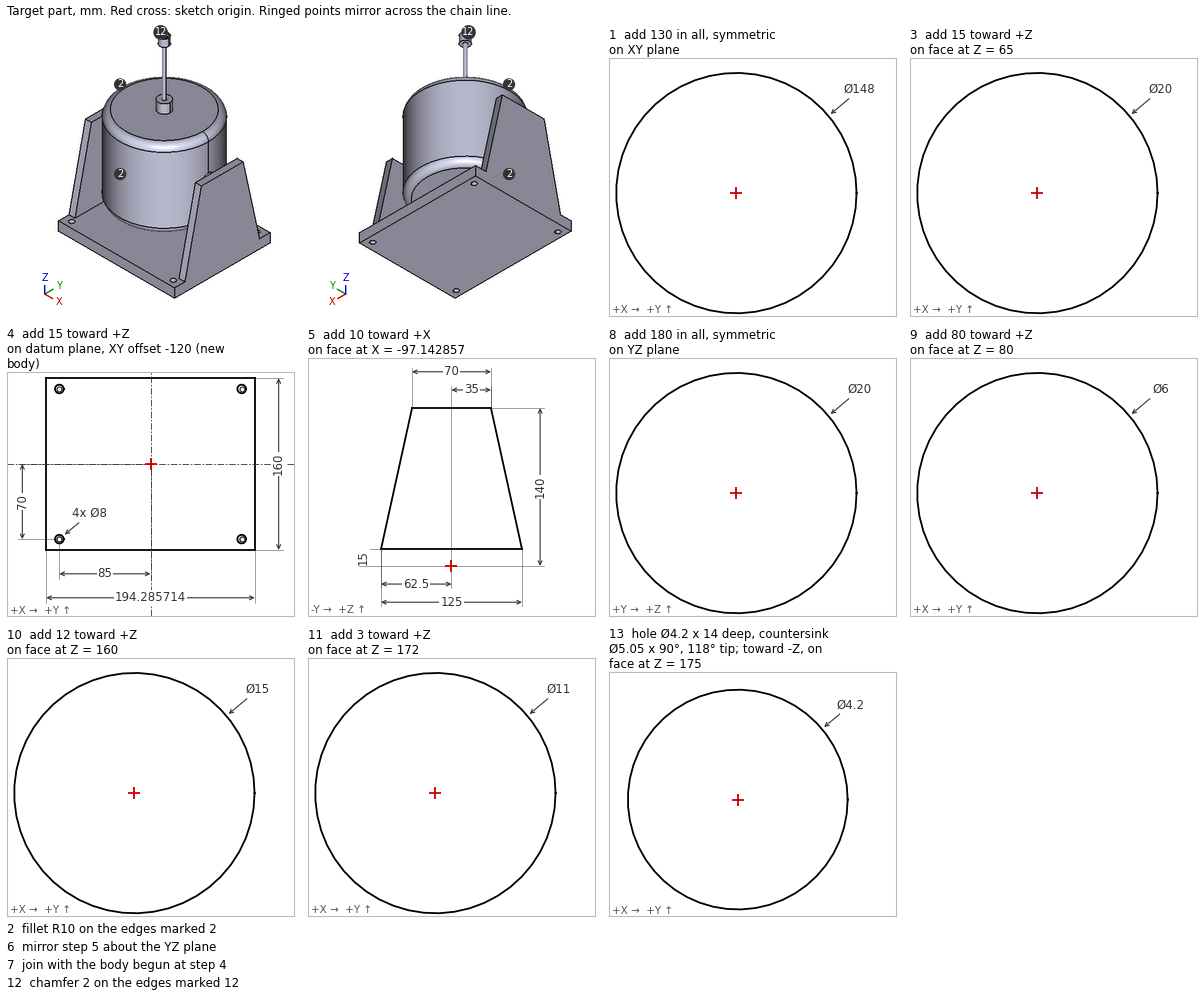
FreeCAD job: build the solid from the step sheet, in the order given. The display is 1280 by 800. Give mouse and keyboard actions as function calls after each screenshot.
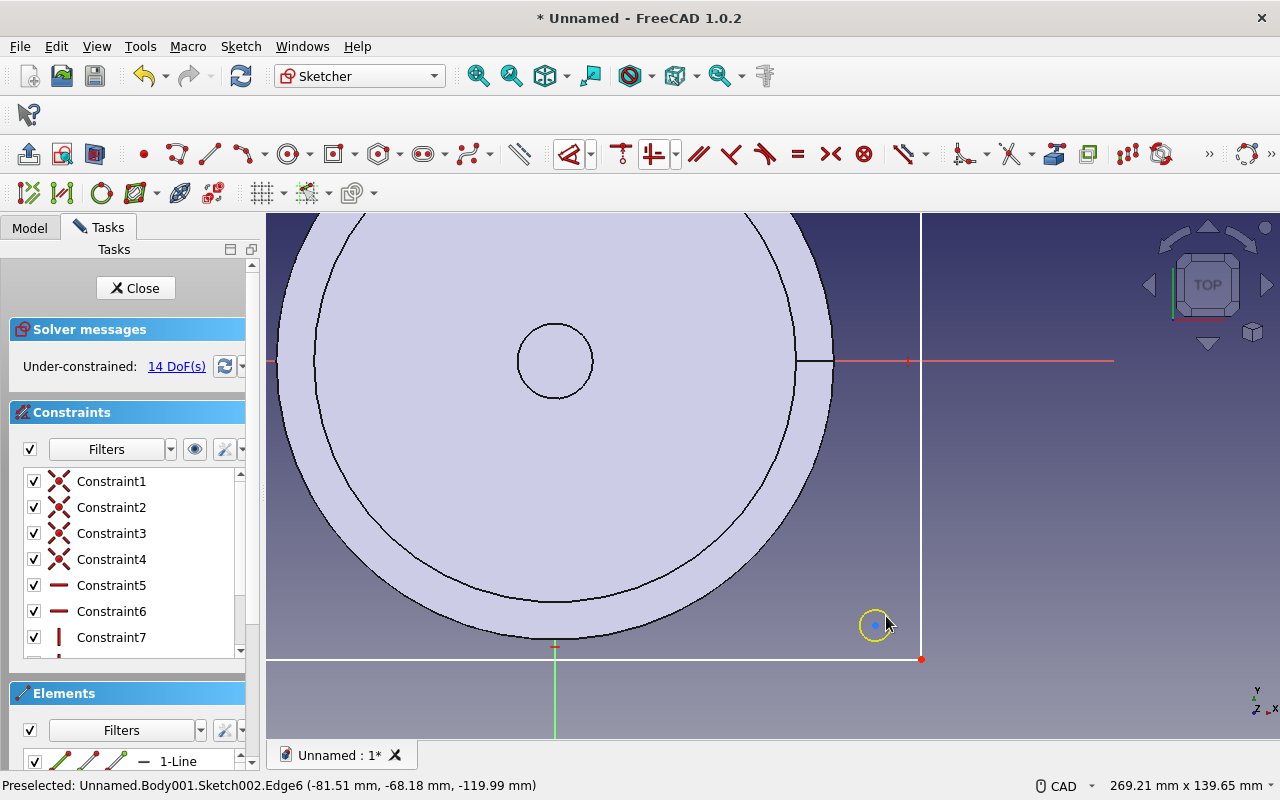
click(886, 615)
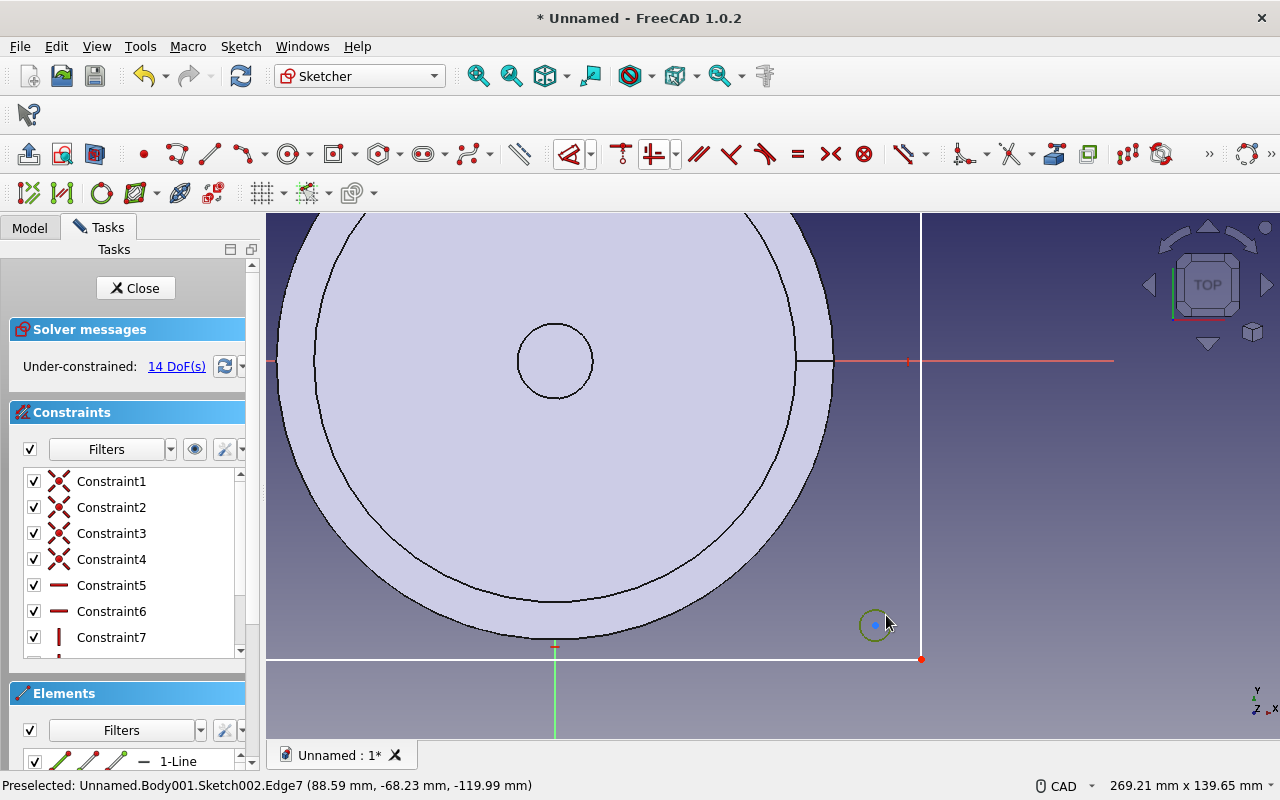
scroll(886, 616, down, 3)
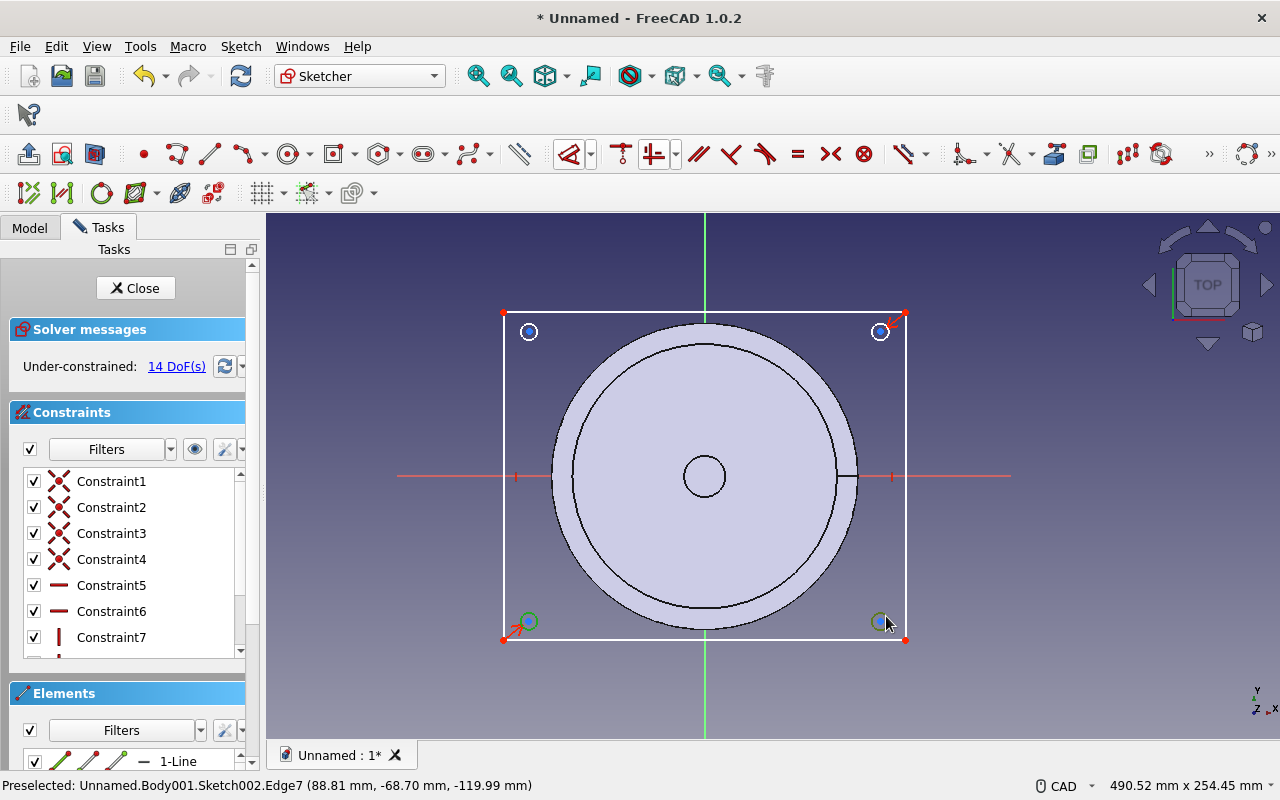
scroll(535, 326, up, 3)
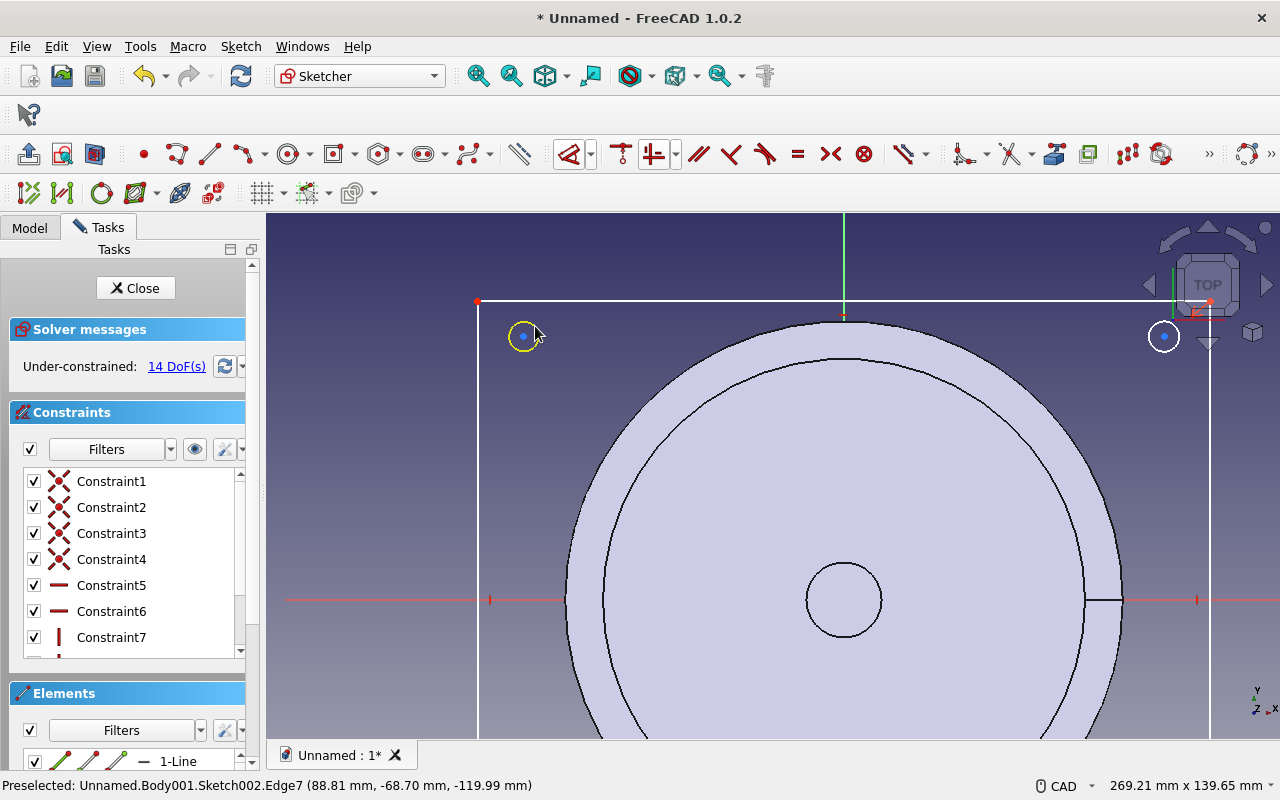
click(534, 326)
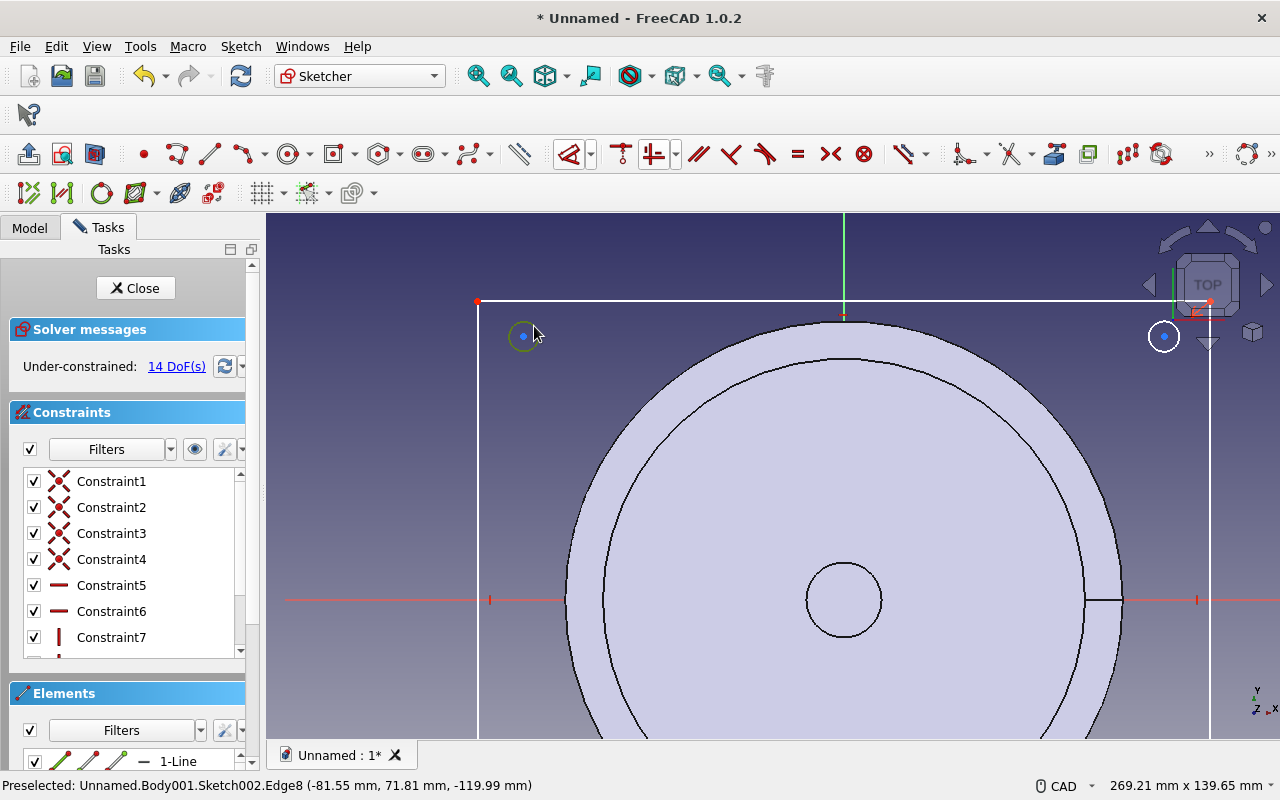
scroll(535, 325, down, 3)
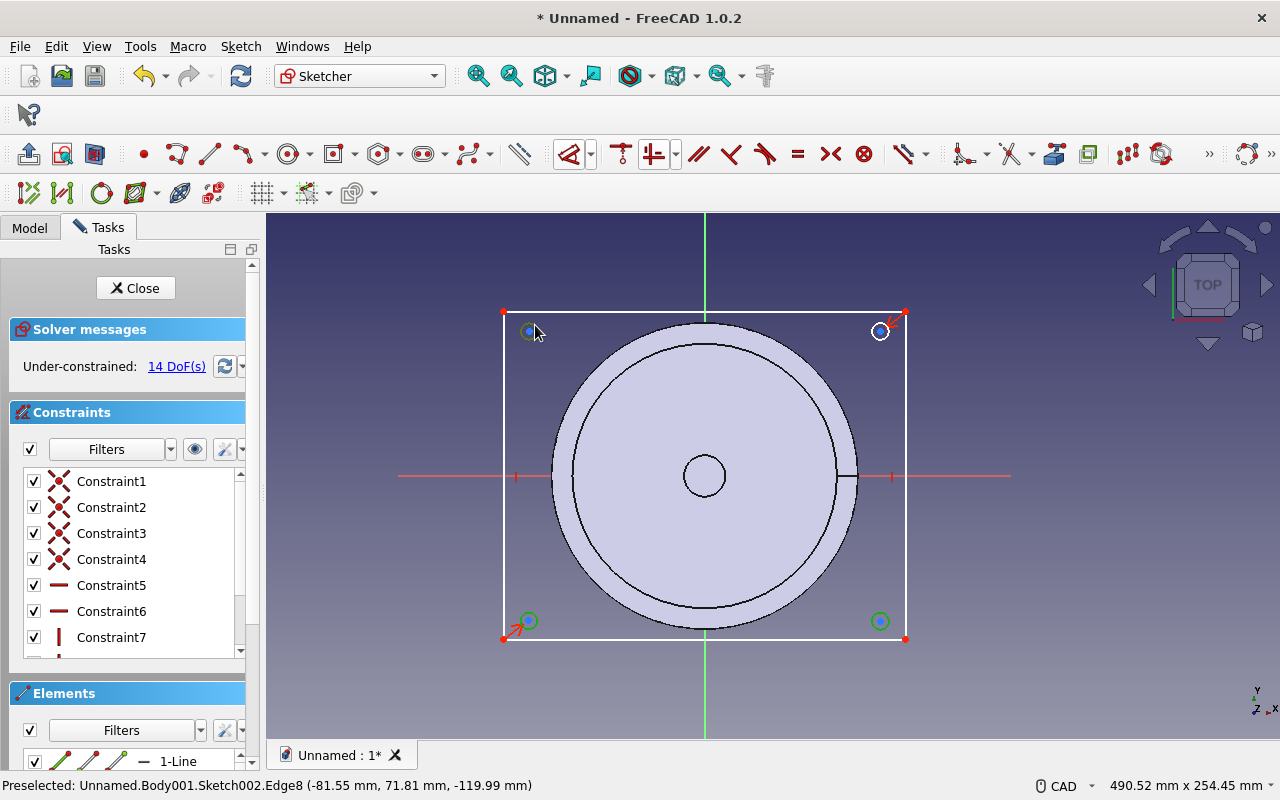
scroll(886, 326, up, 3)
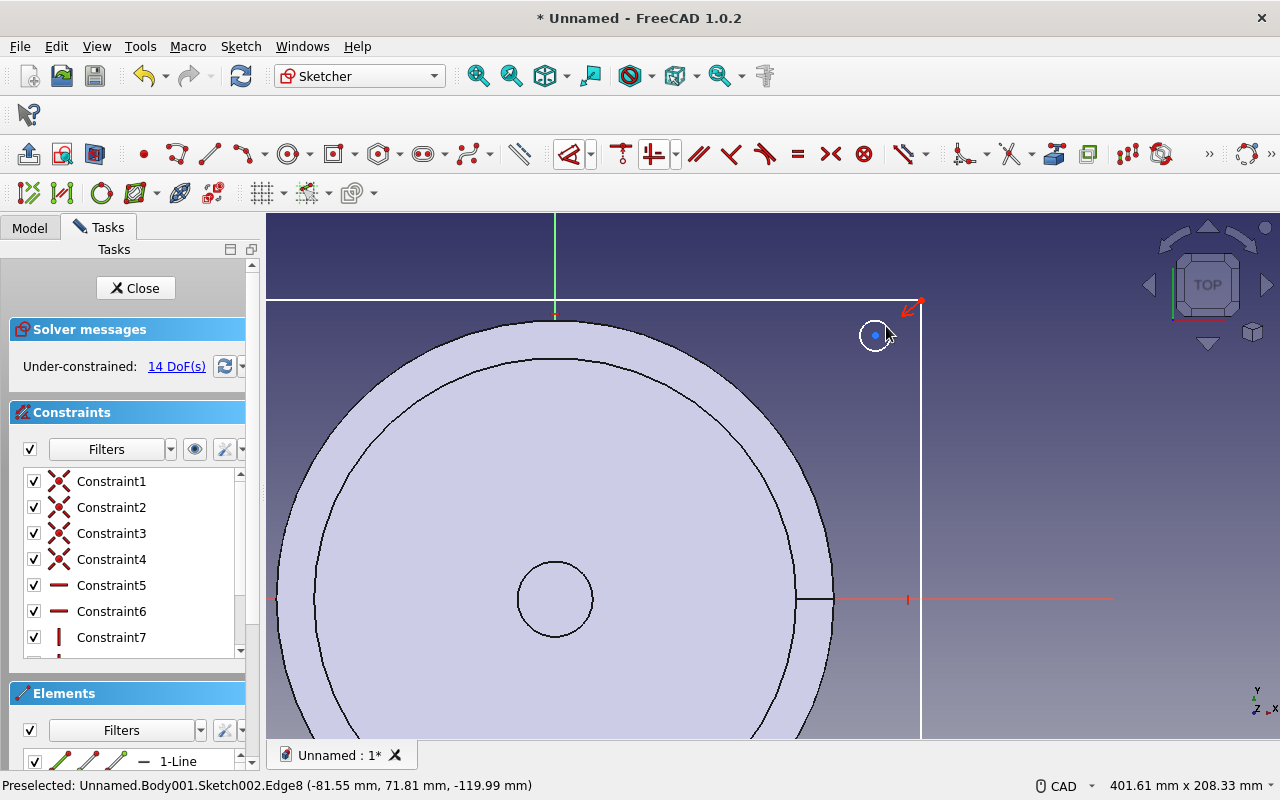
click(886, 325)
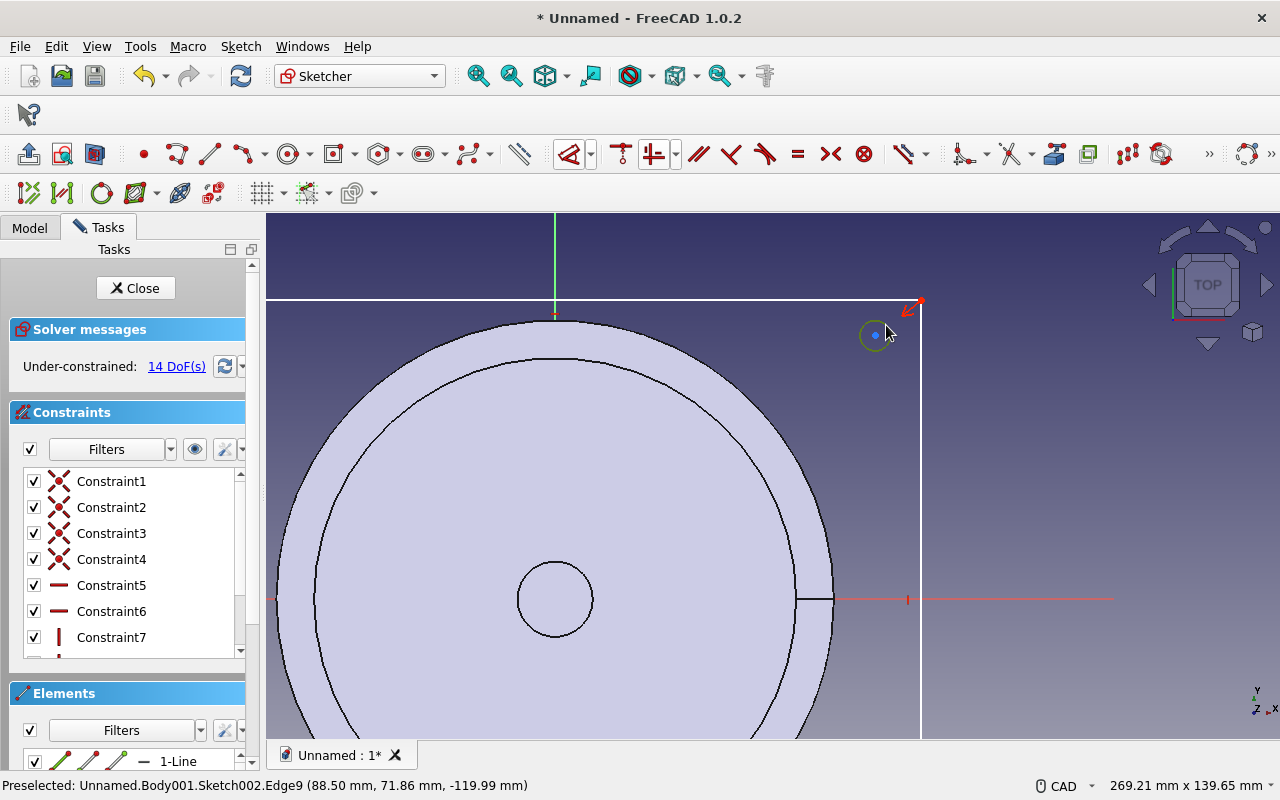
key(e)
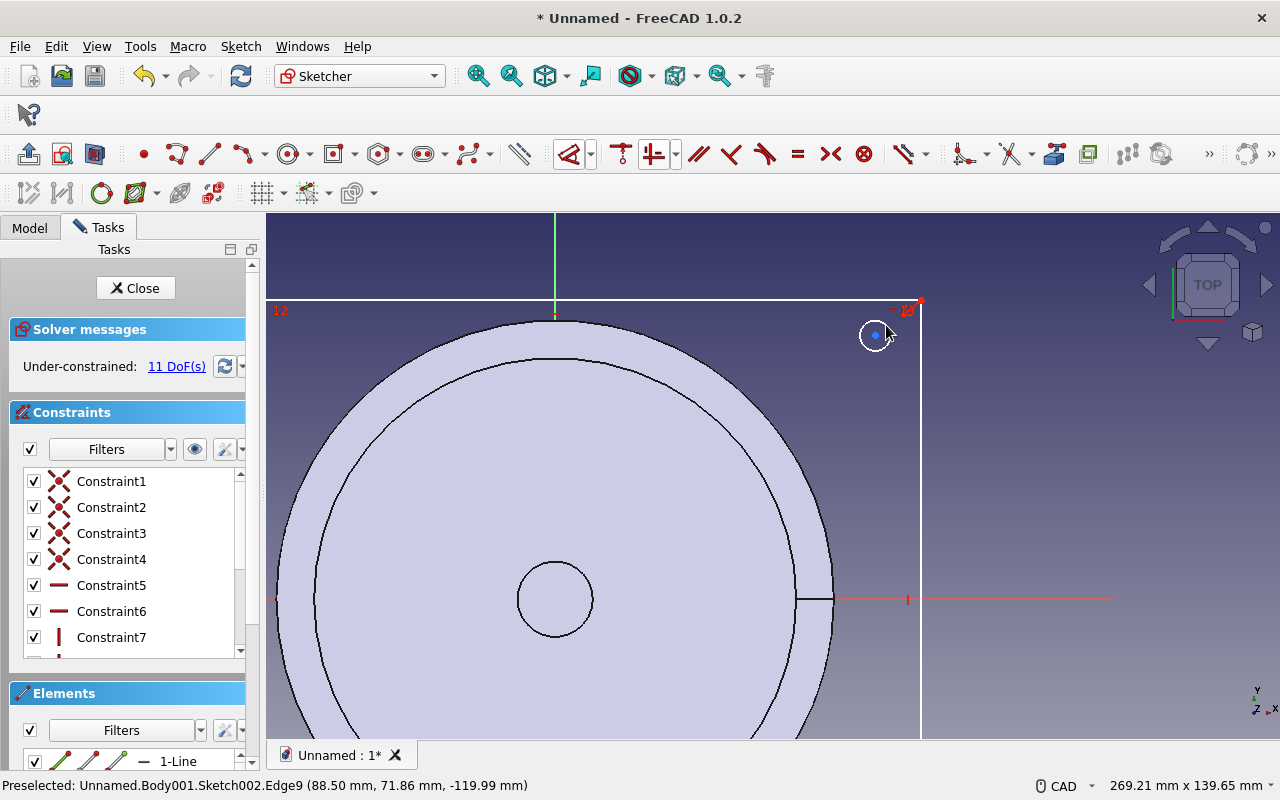
scroll(886, 326, down, 3)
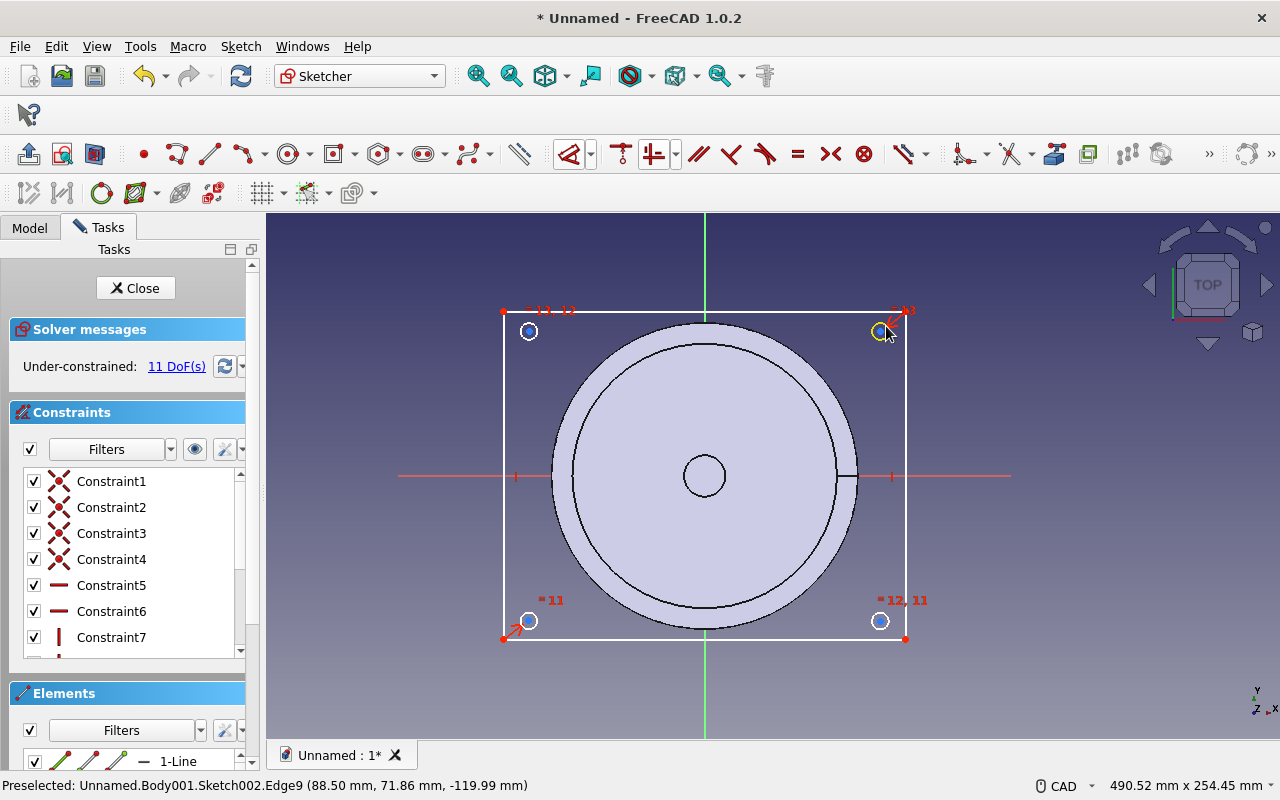
click(529, 621)